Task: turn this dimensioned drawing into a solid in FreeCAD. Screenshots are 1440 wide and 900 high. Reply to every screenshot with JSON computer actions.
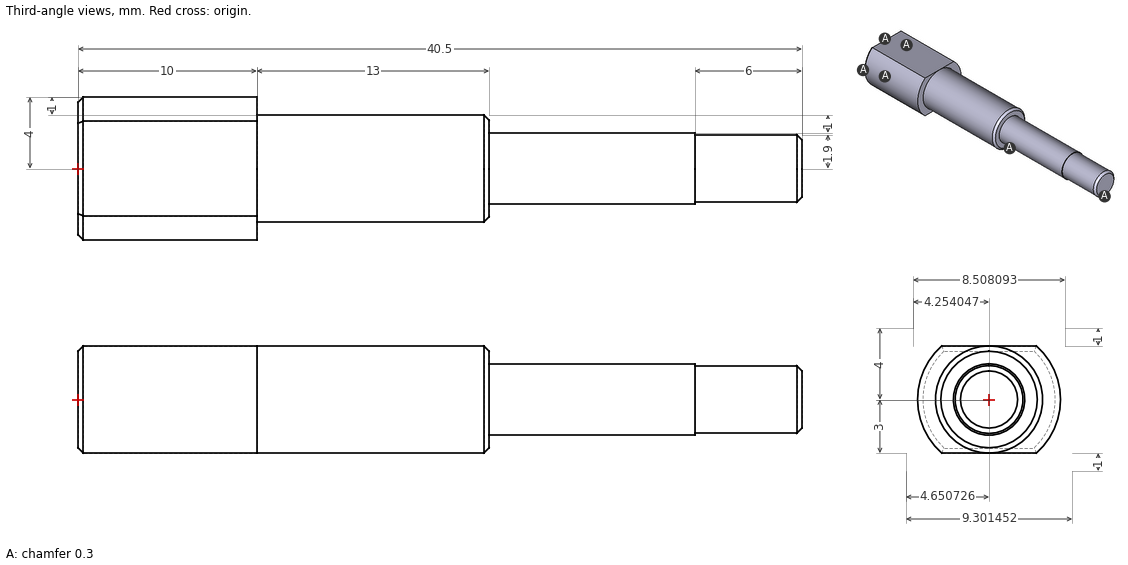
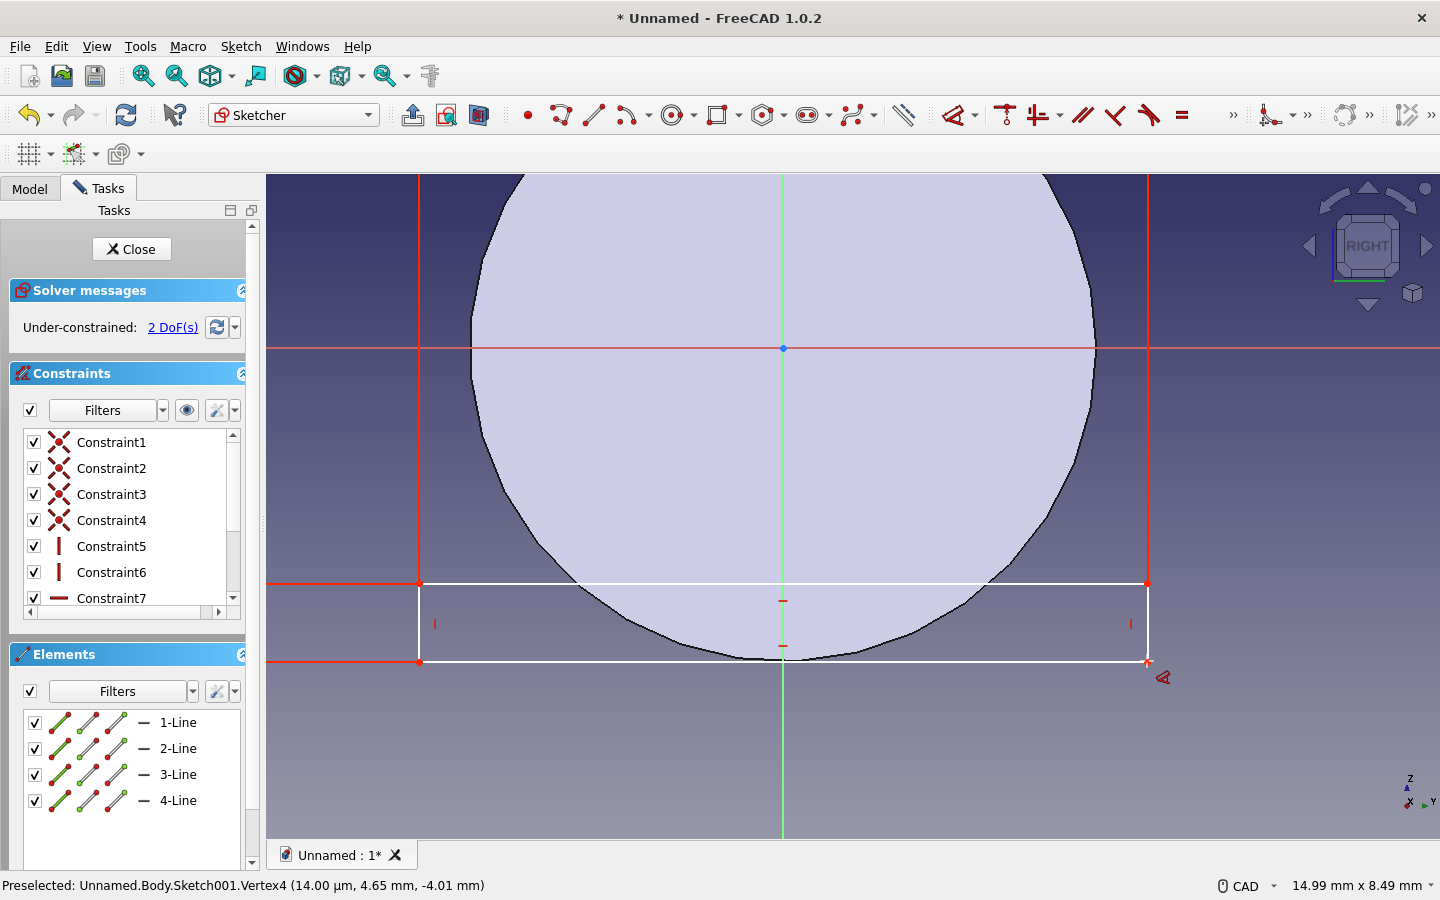
{"action": "left_click", "coordinate": [419, 584]}
{"action": "left_click", "coordinate": [385, 466]}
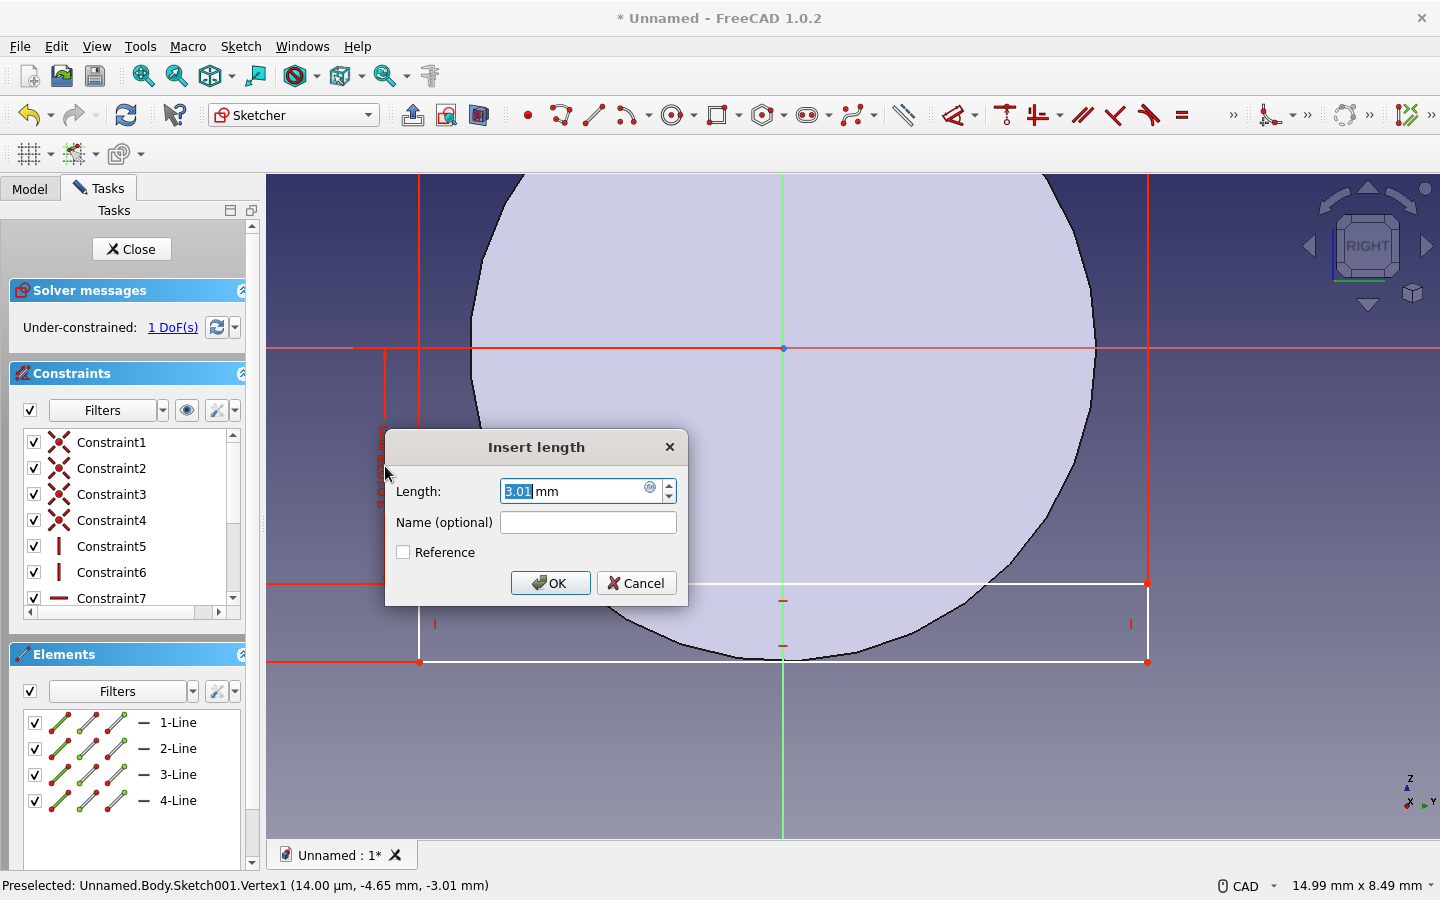
{"action": "type", "text": "3"}
{"action": "key", "text": "Return"}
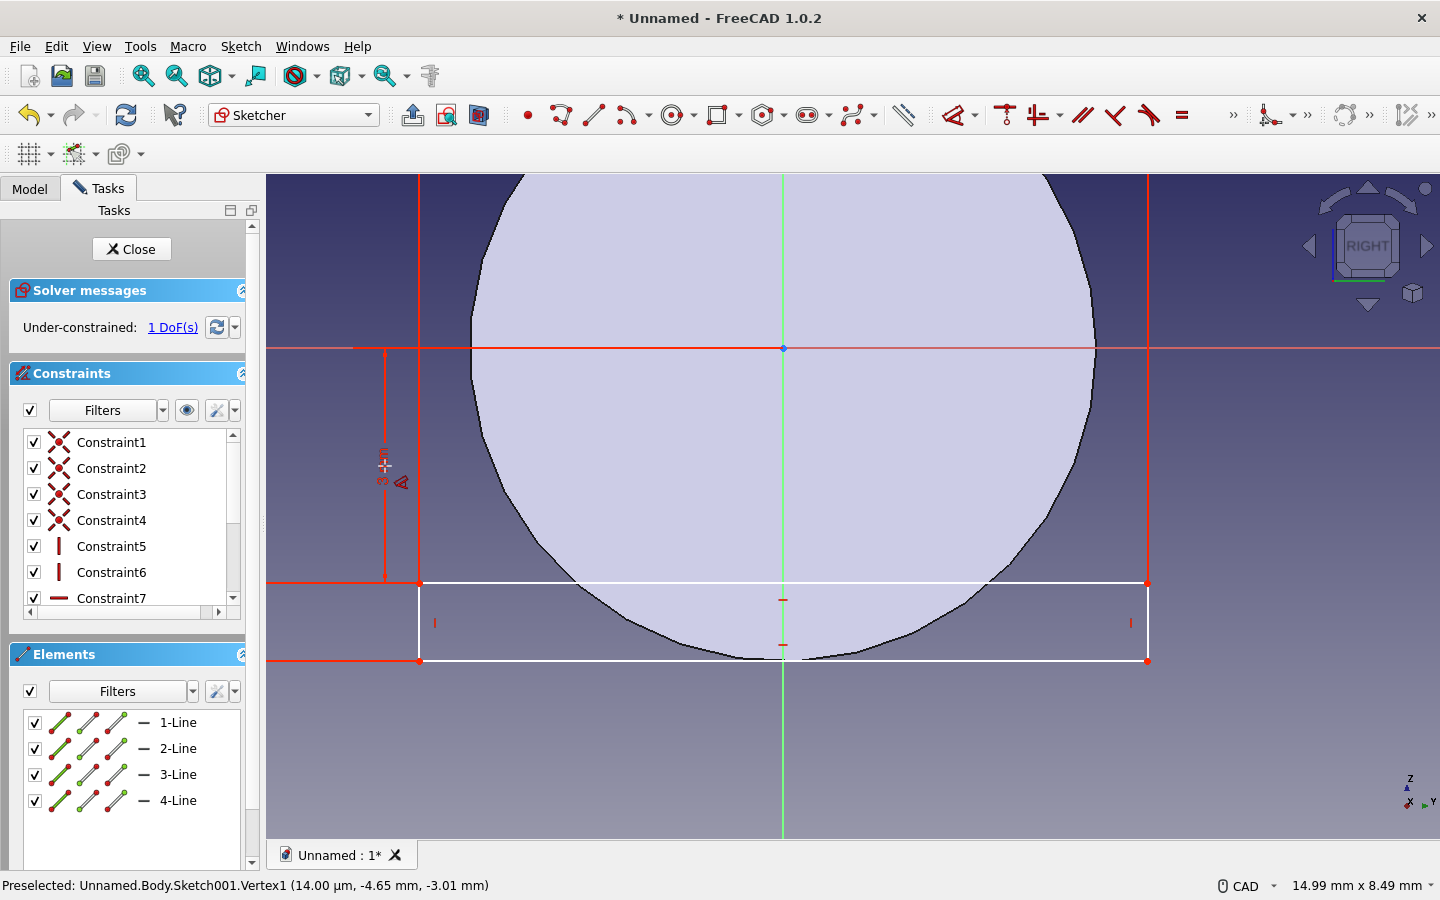
{"action": "left_click", "coordinate": [419, 583]}
{"action": "left_click", "coordinate": [601, 314]}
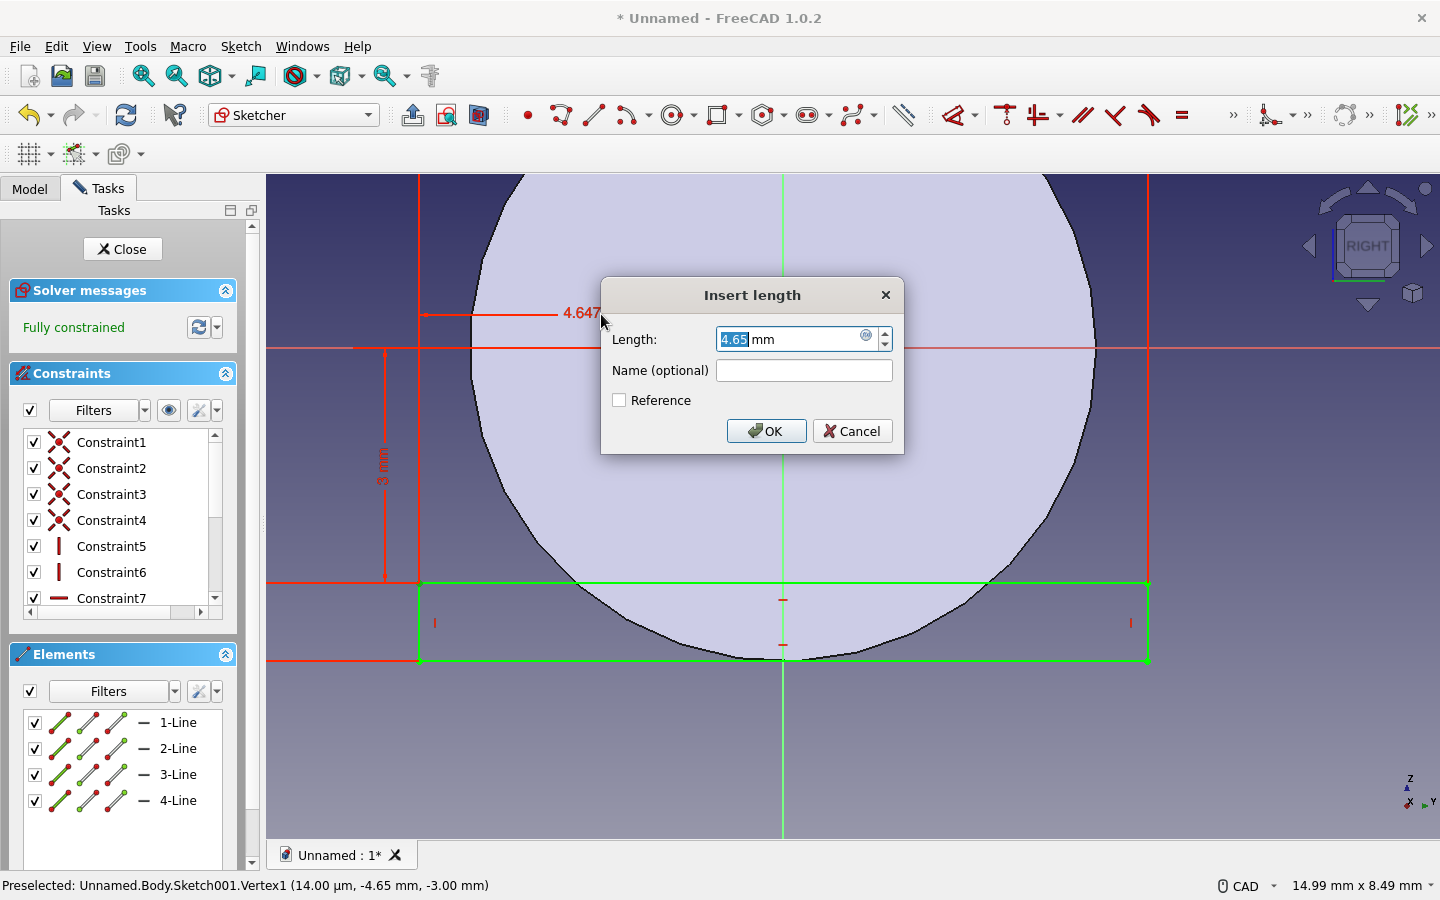
{"action": "type", "text": "4.650726"}
{"action": "key", "text": "Return"}
{"action": "key", "text": "Escape"}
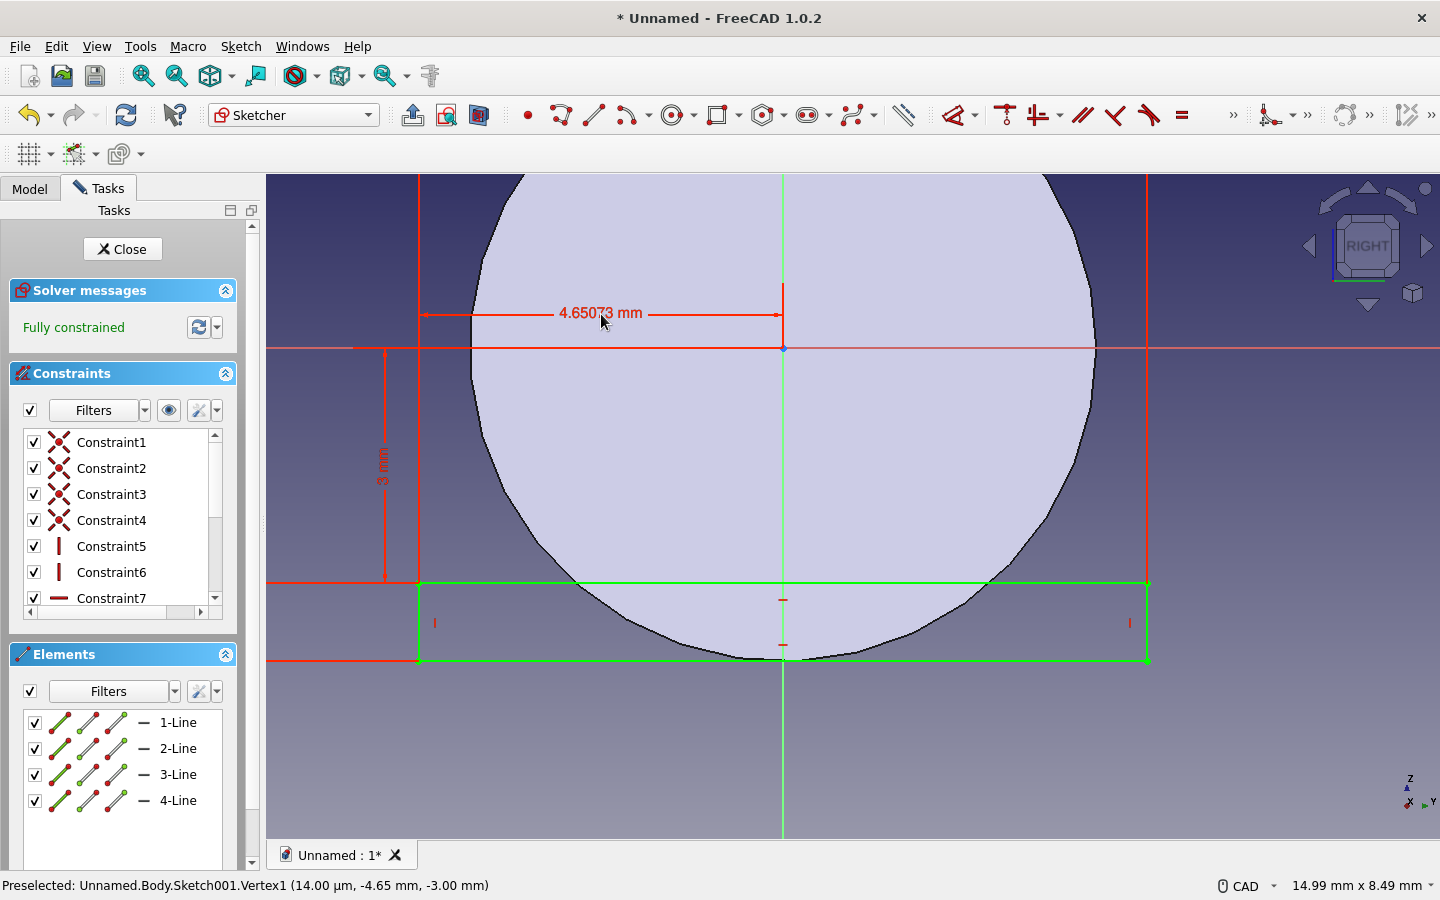
{"action": "left_click", "coordinate": [123, 249]}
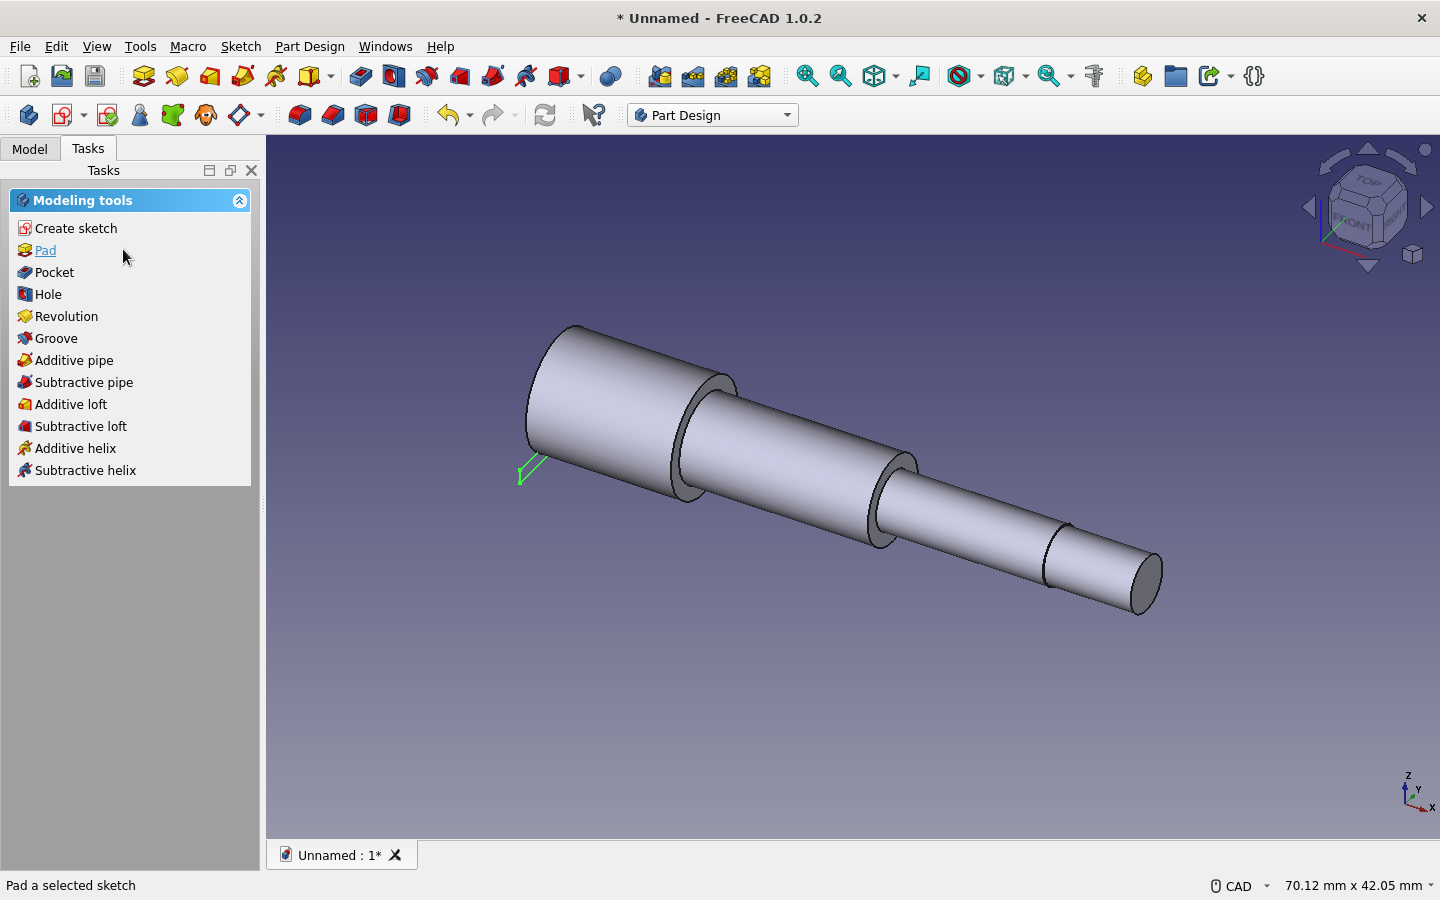
{"action": "left_click", "coordinate": [361, 76]}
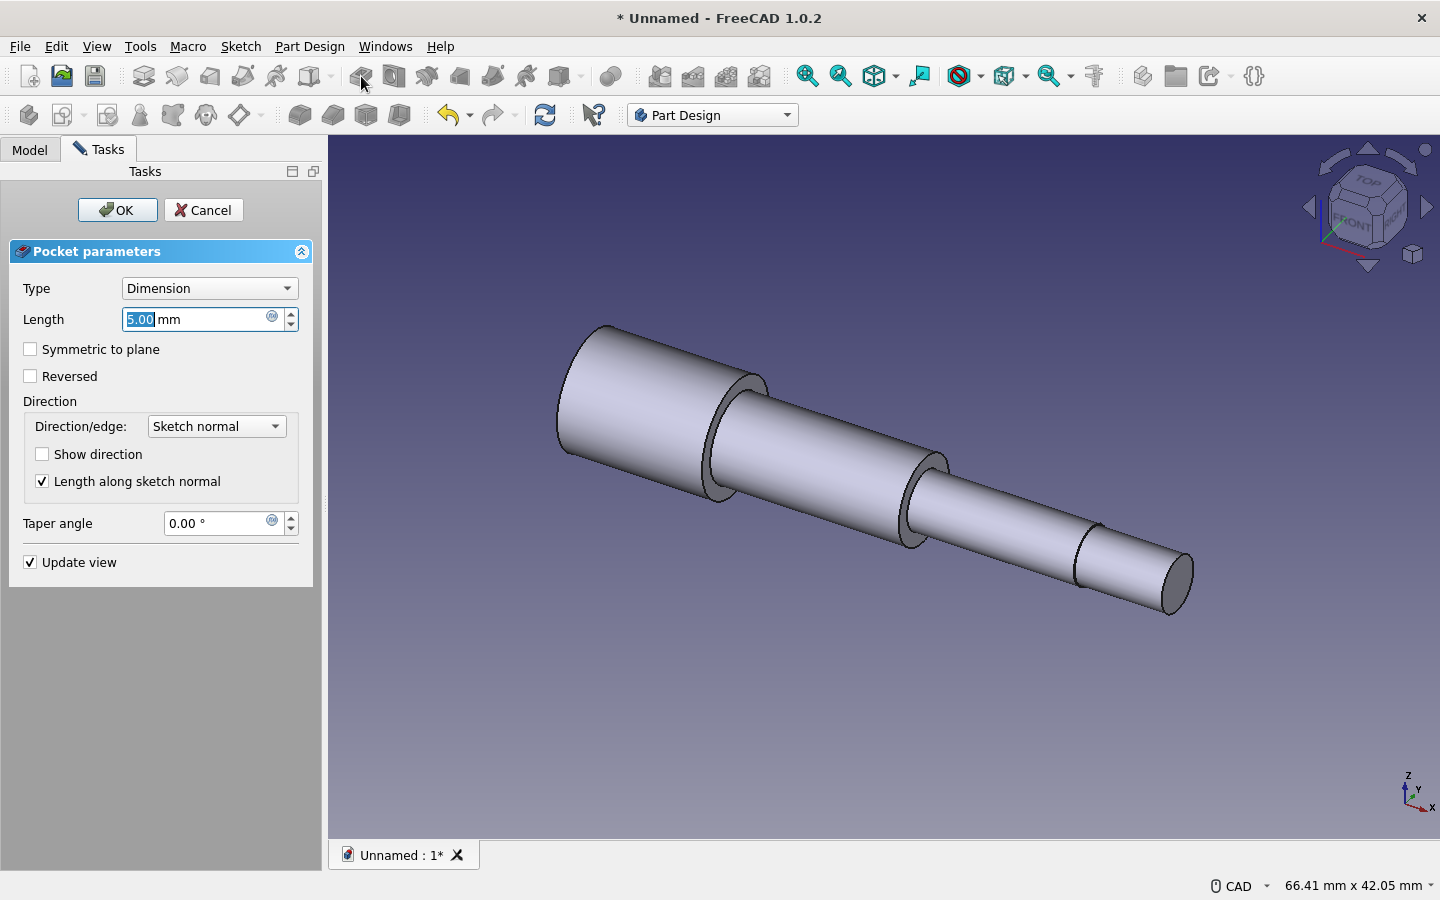
{"action": "left_click", "coordinate": [210, 288]}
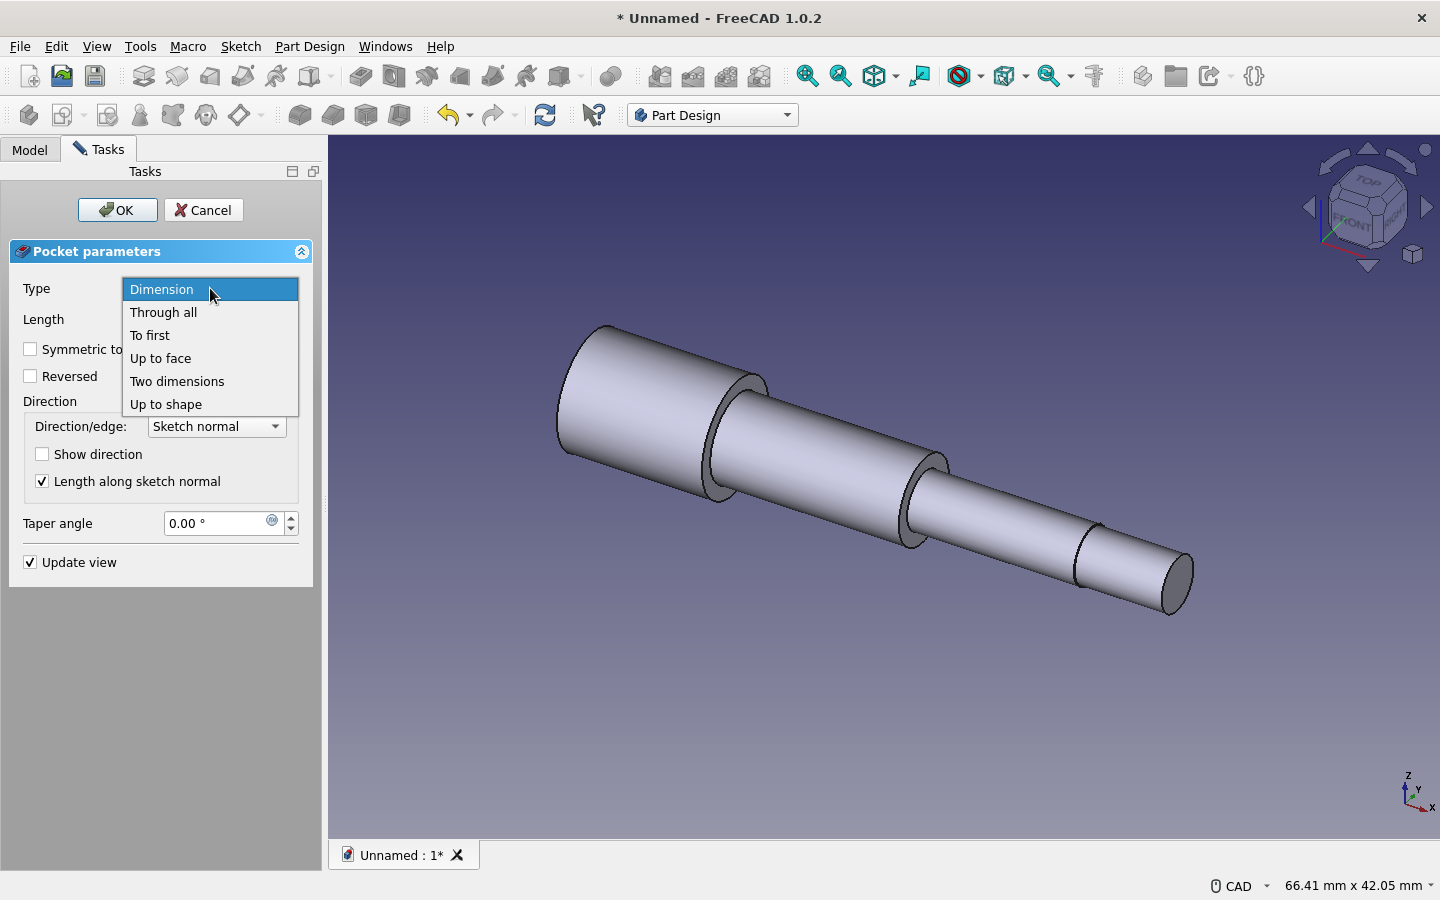
{"action": "left_click", "coordinate": [208, 336]}